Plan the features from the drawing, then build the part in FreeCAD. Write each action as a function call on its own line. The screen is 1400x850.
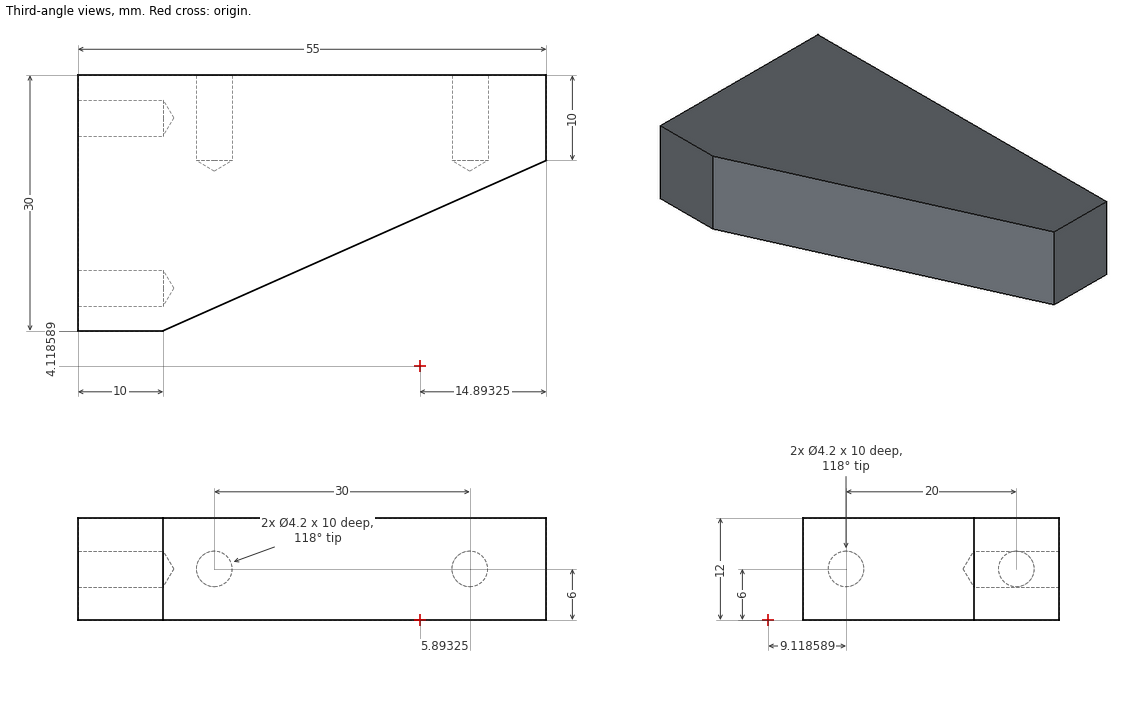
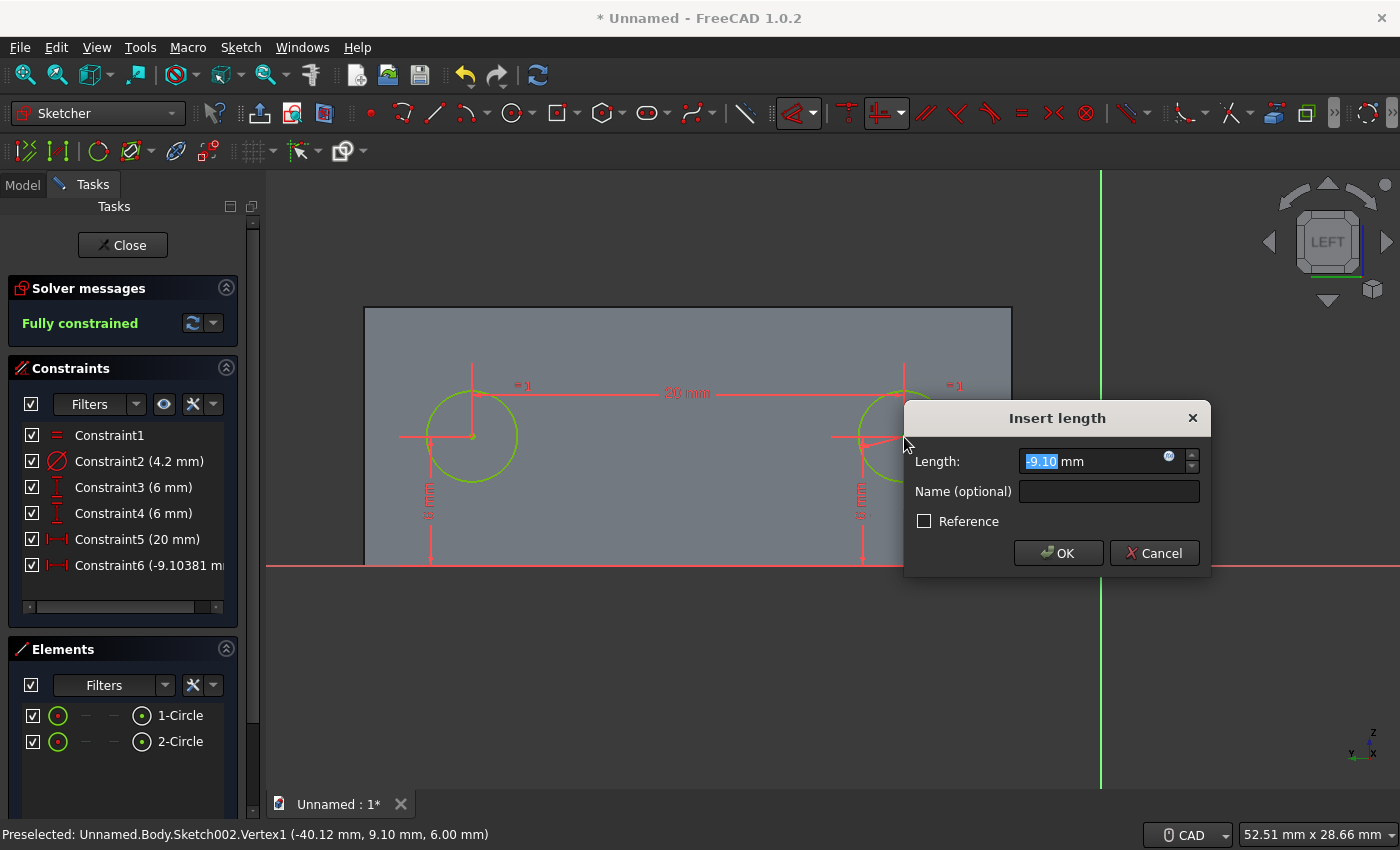
text(-9.118589)
key(Return)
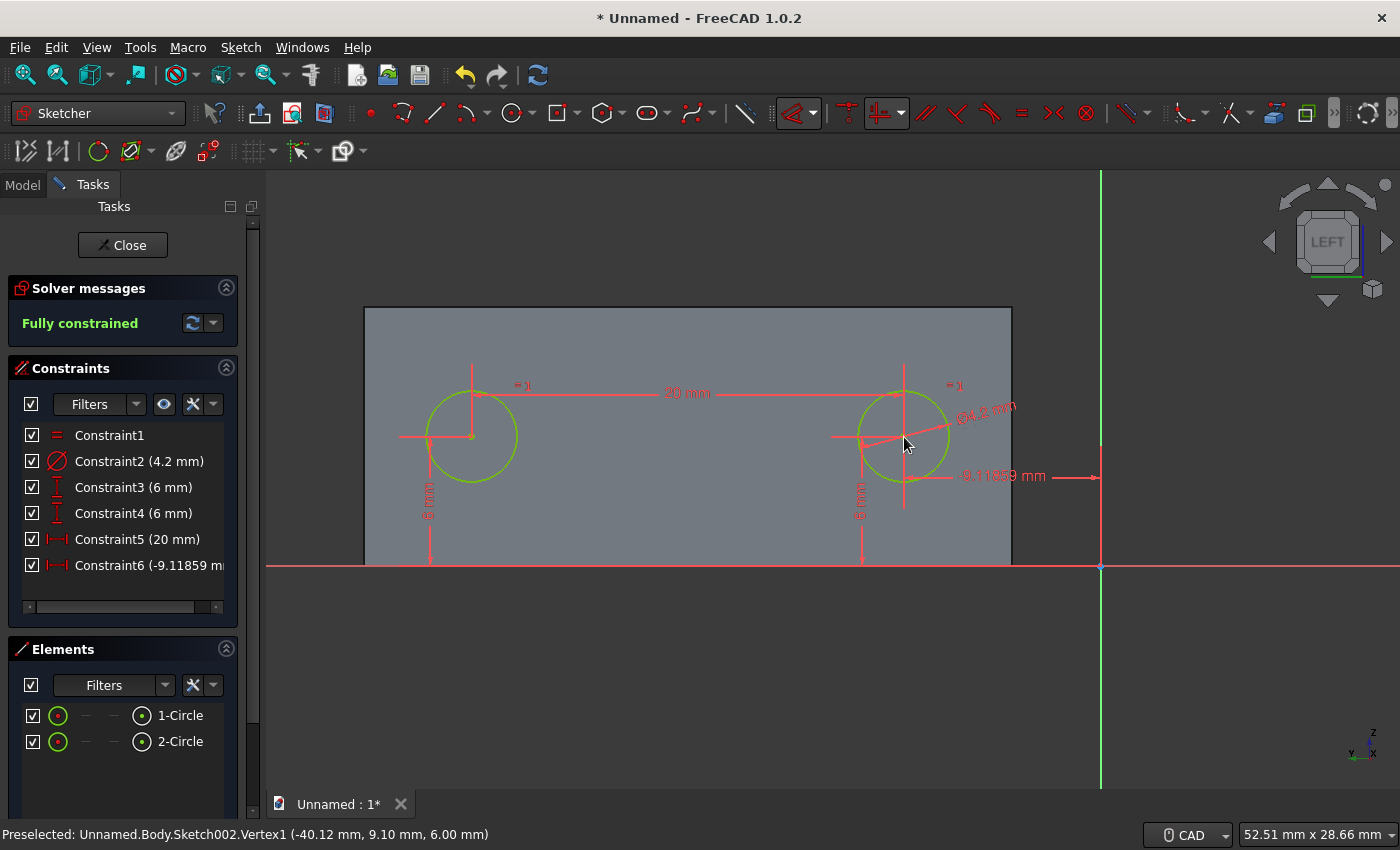
click(123, 245)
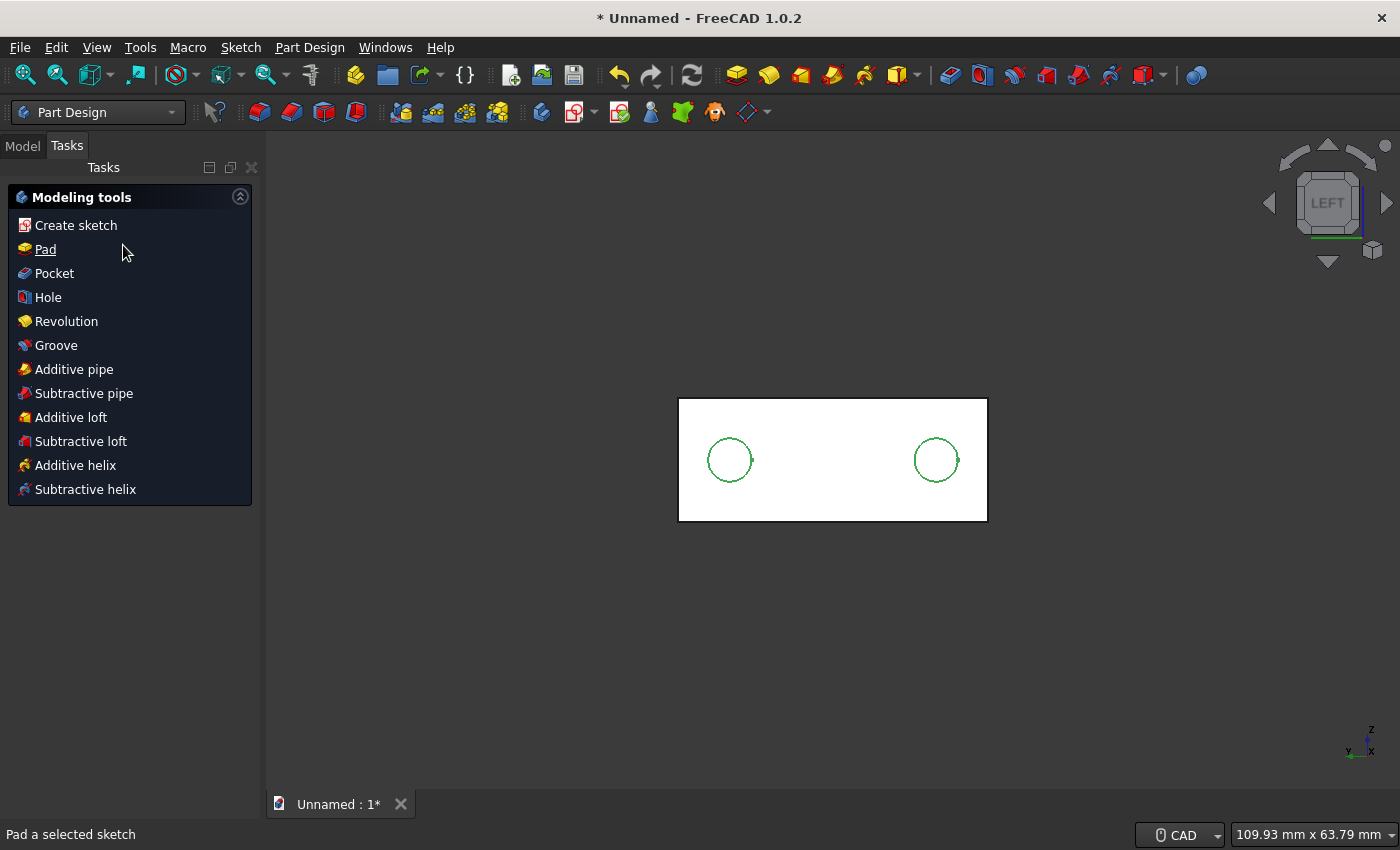
click(984, 76)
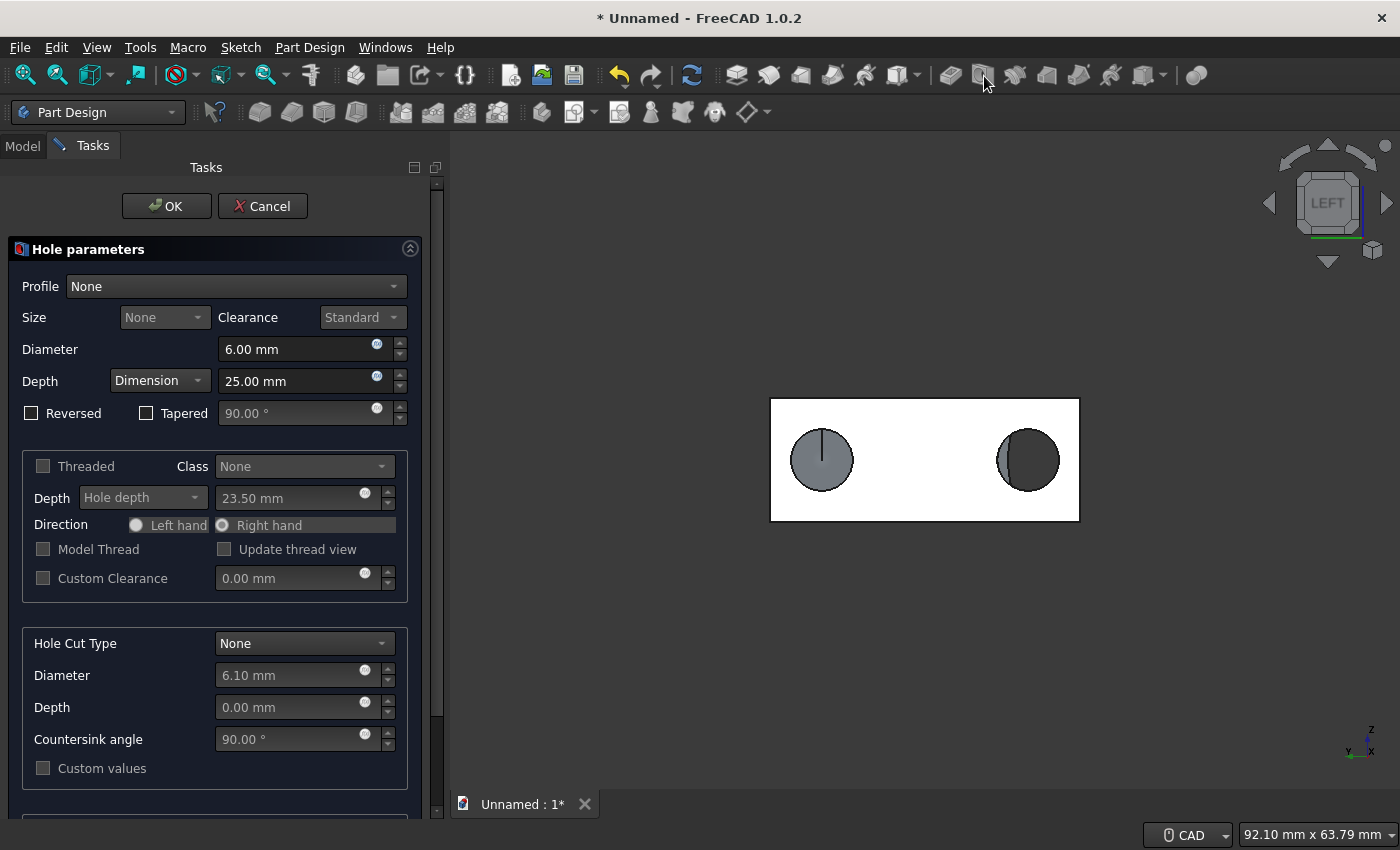
triple_click(305, 349)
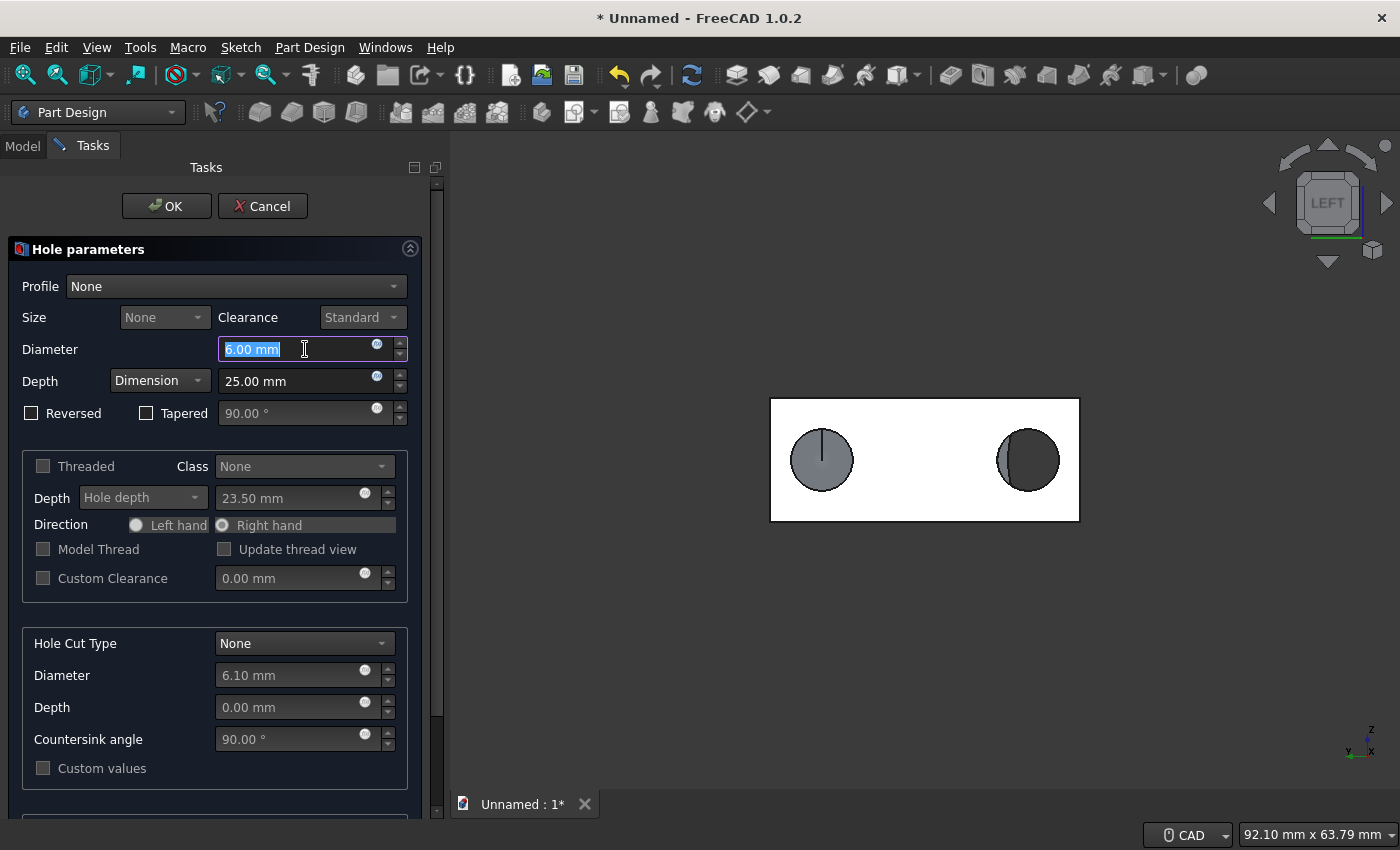
text(4.2)
key(Tab)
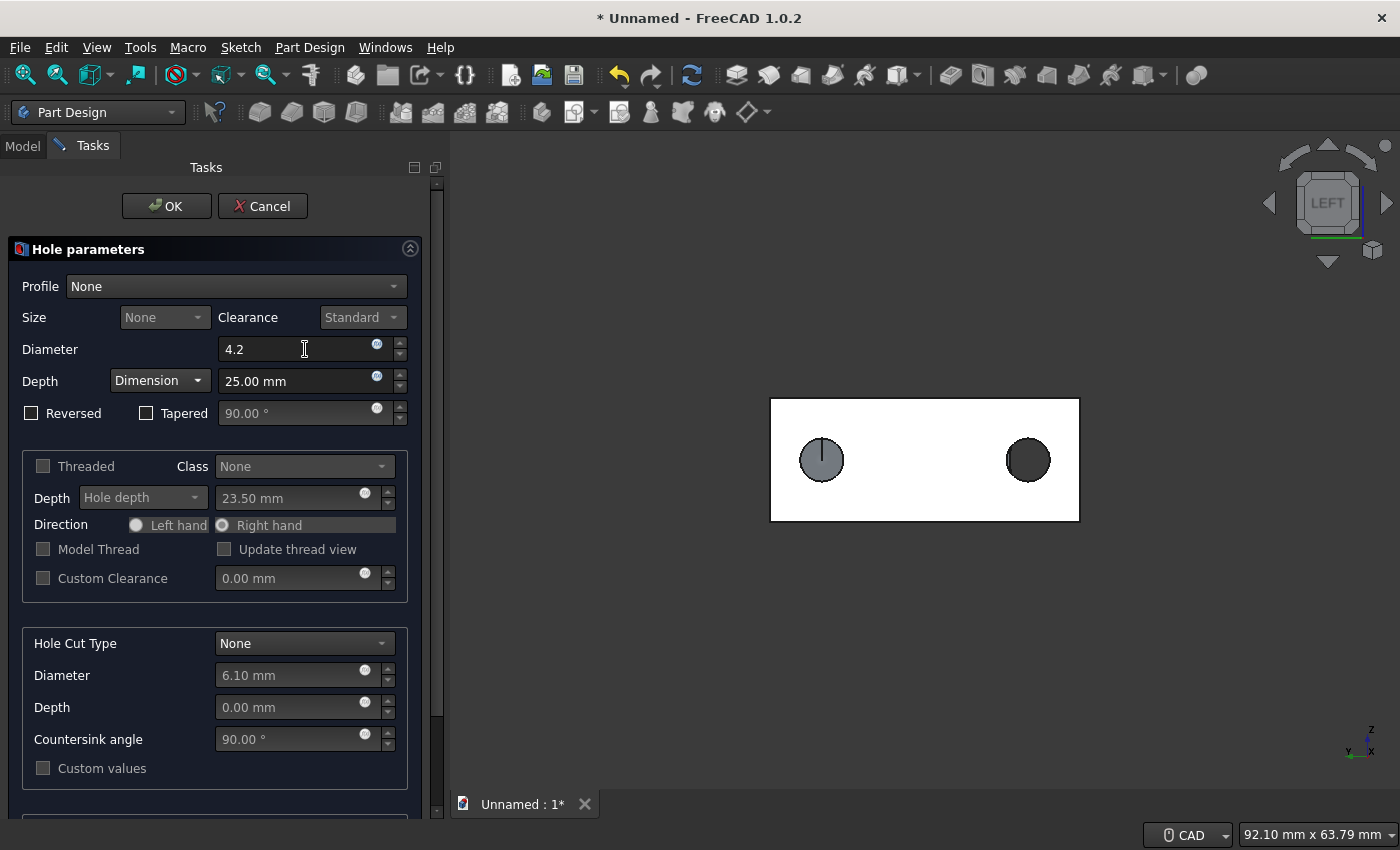
triple_click(305, 381)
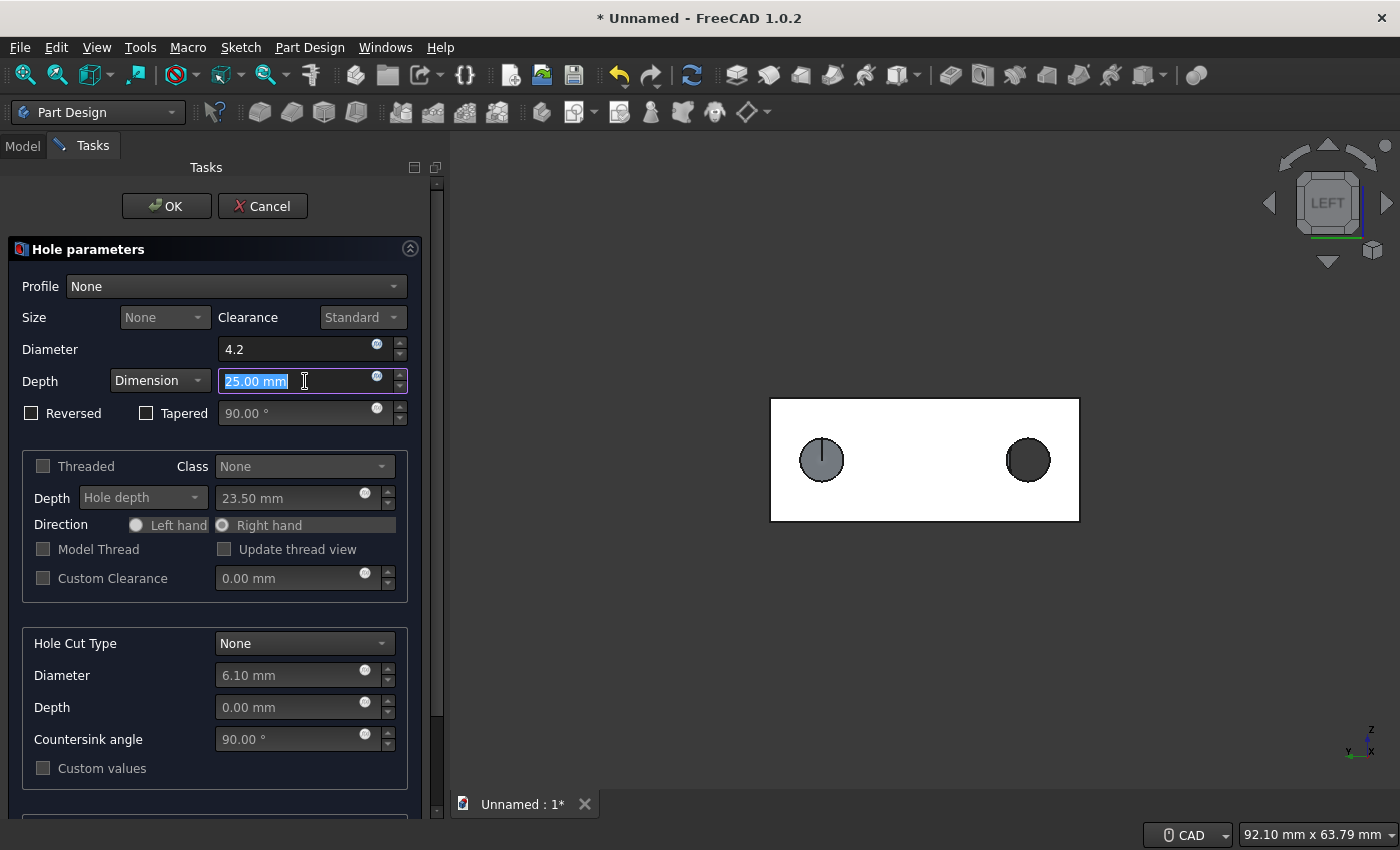
text(10)
key(Tab)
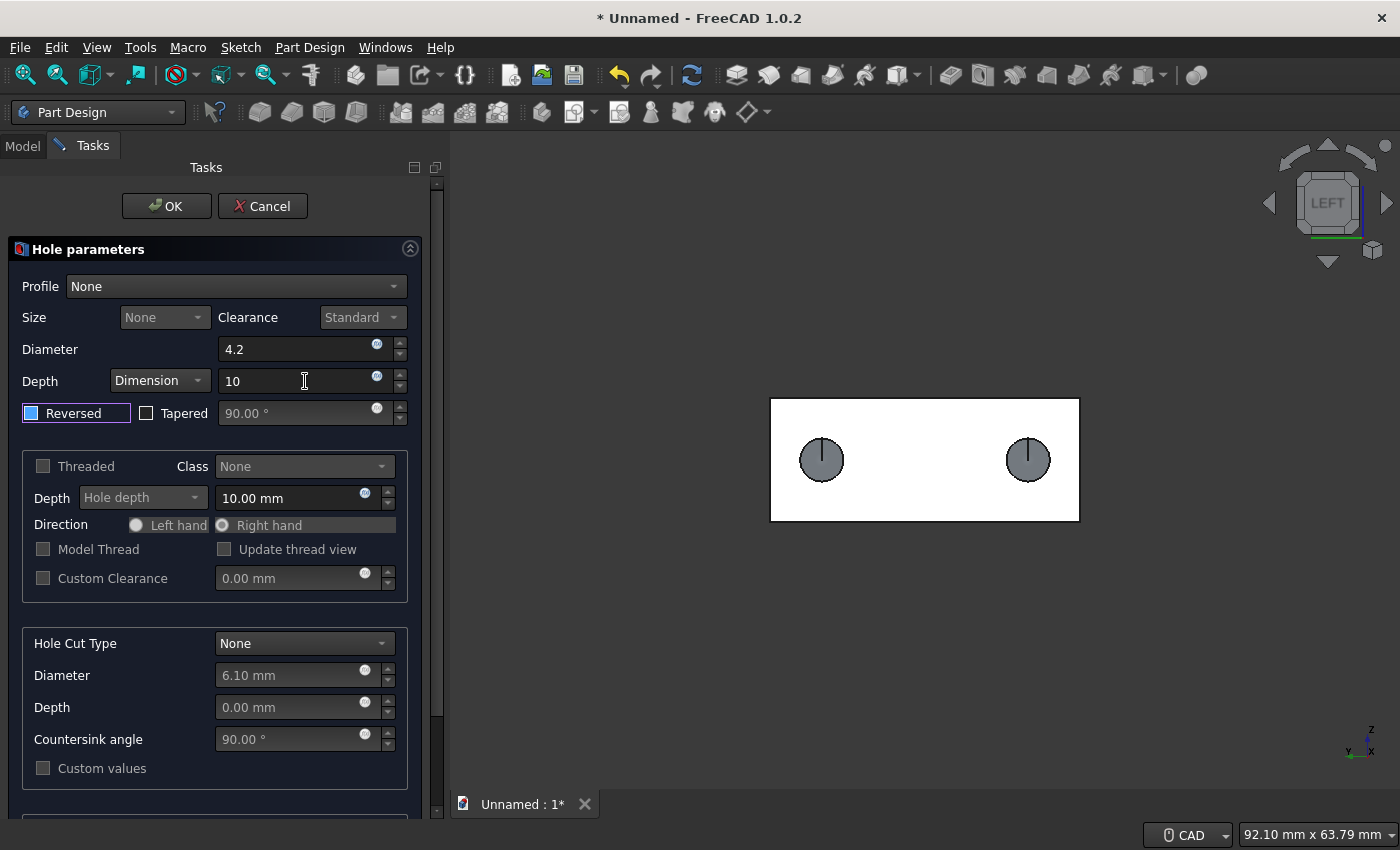
click(167, 206)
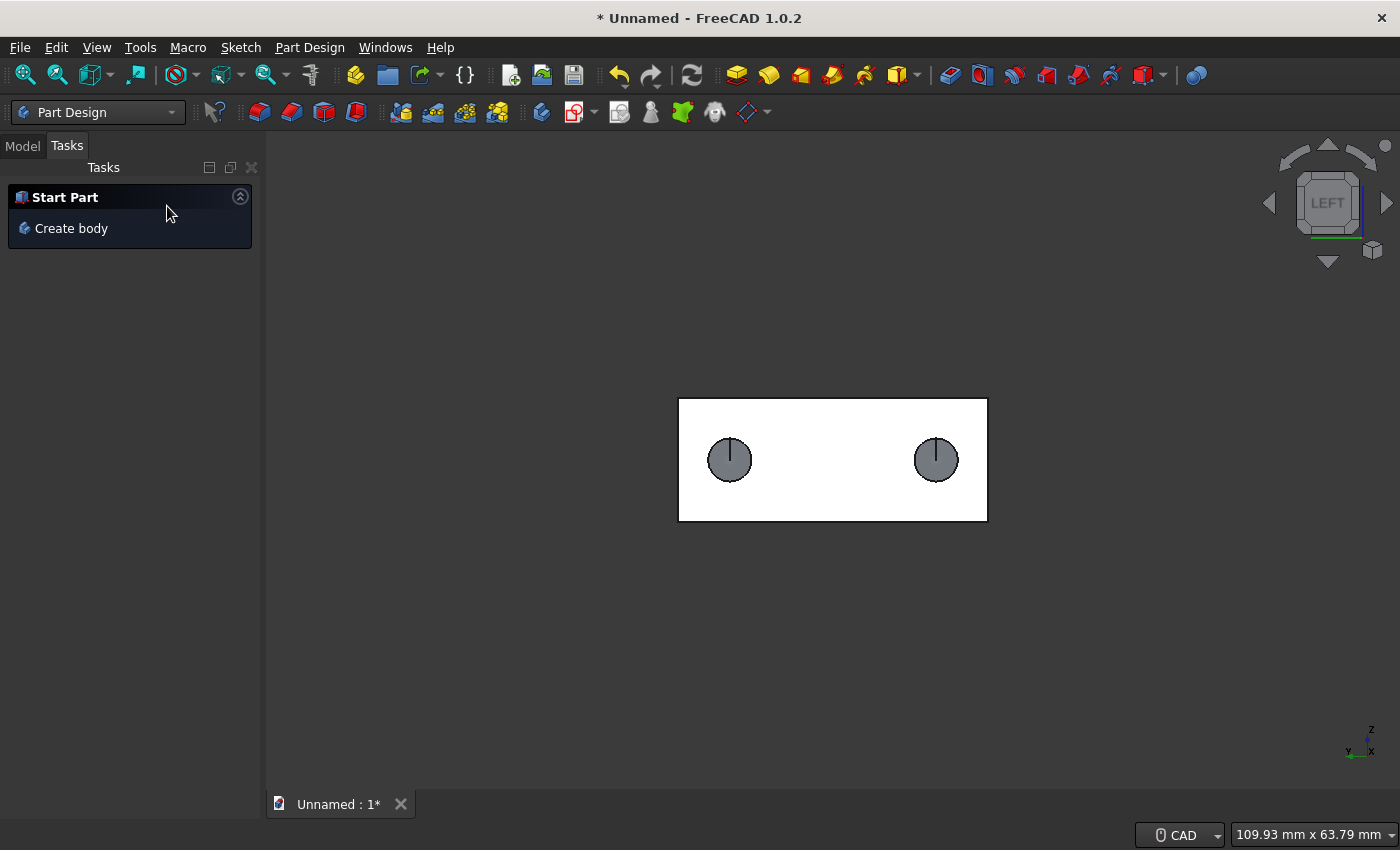
key(0)